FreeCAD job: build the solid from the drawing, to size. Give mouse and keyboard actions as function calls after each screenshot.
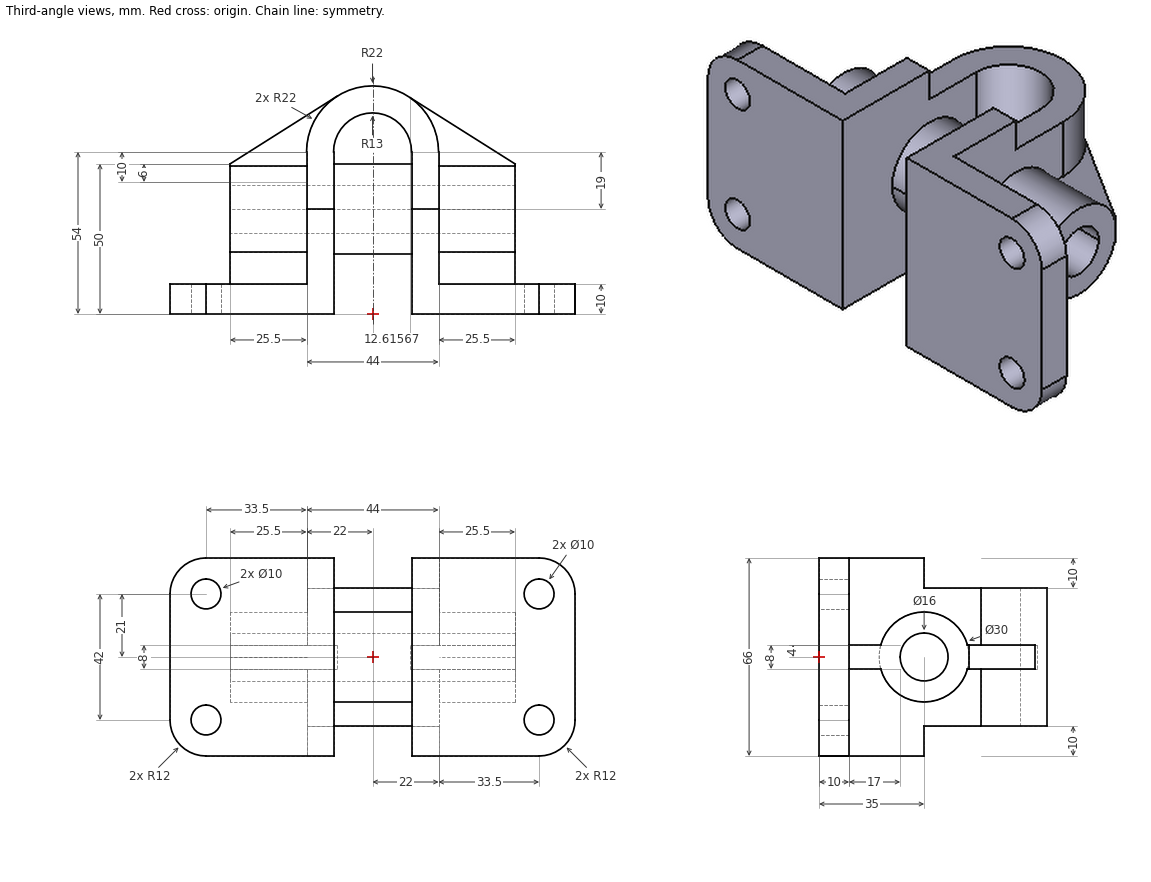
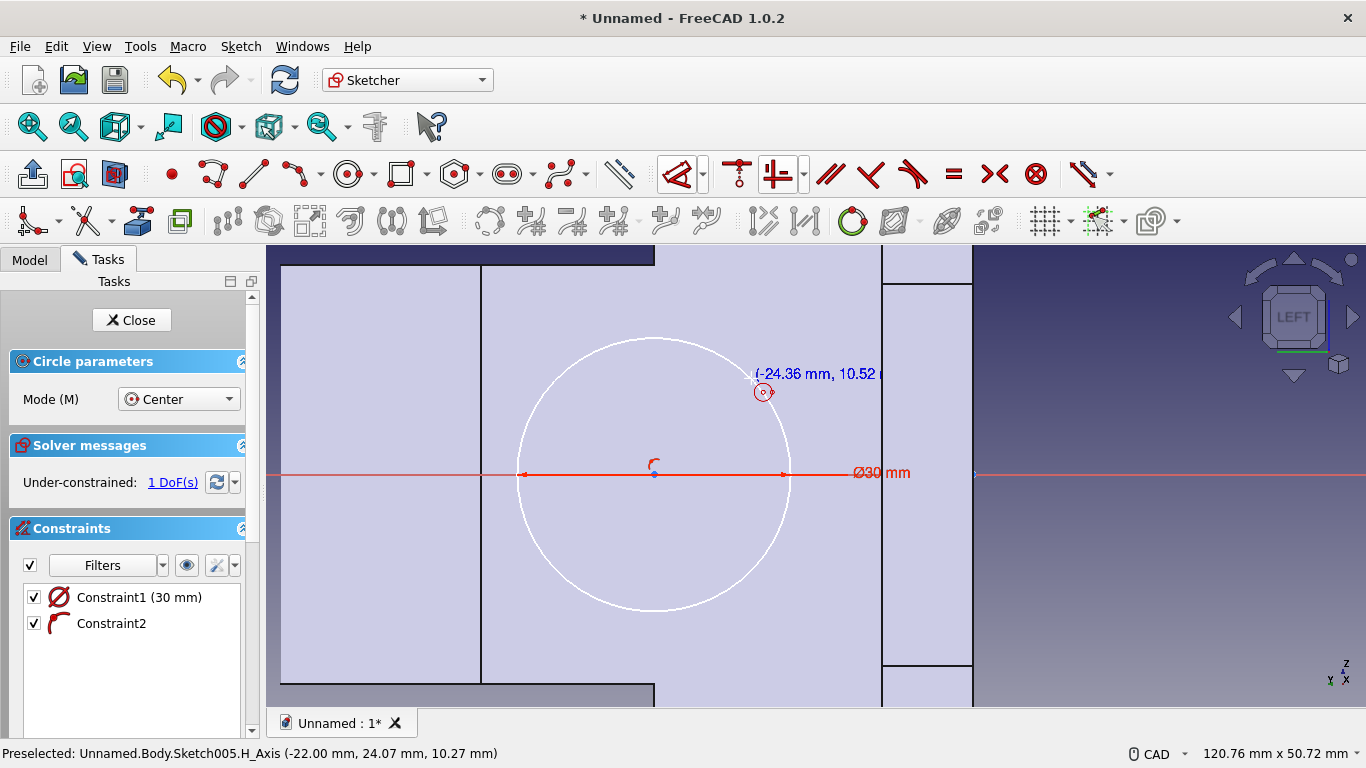
click(654, 475)
move(706, 423)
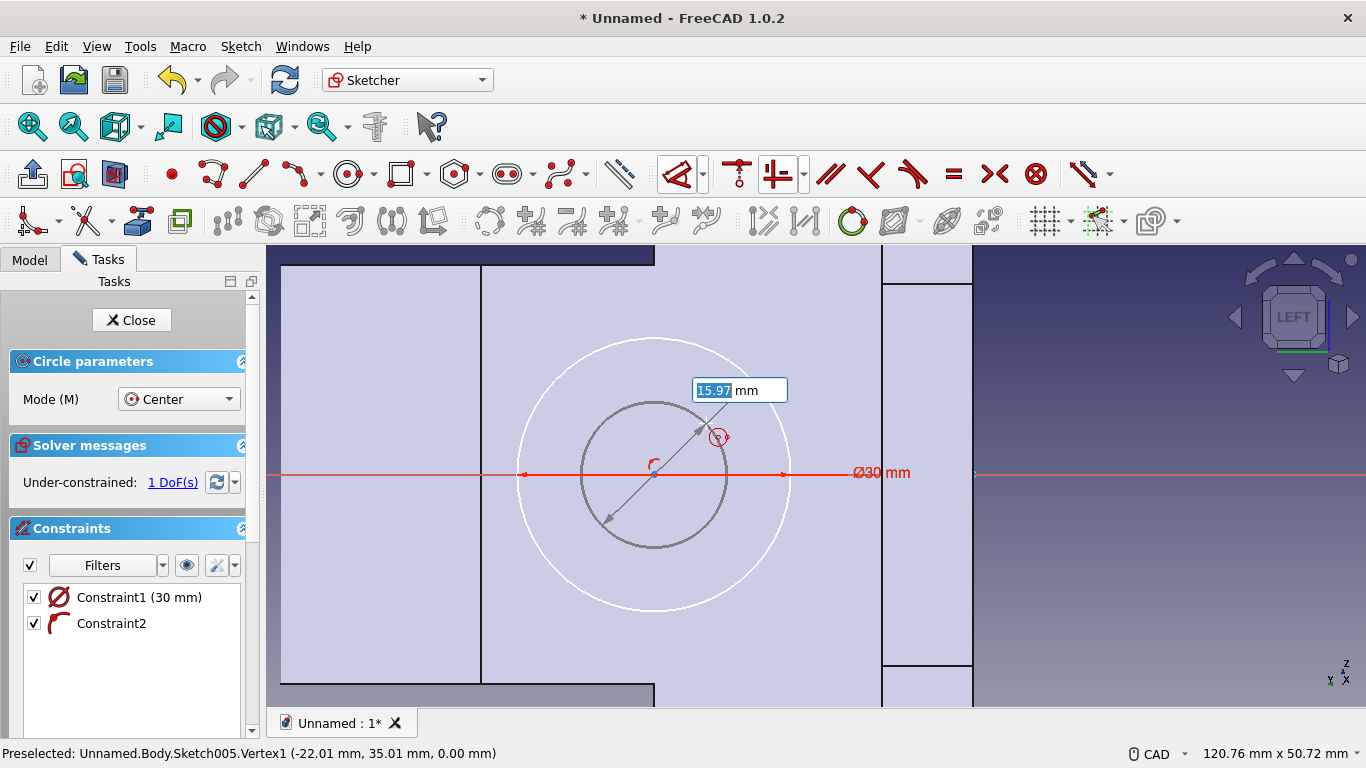
text(16)
key(Return)
key(Escape)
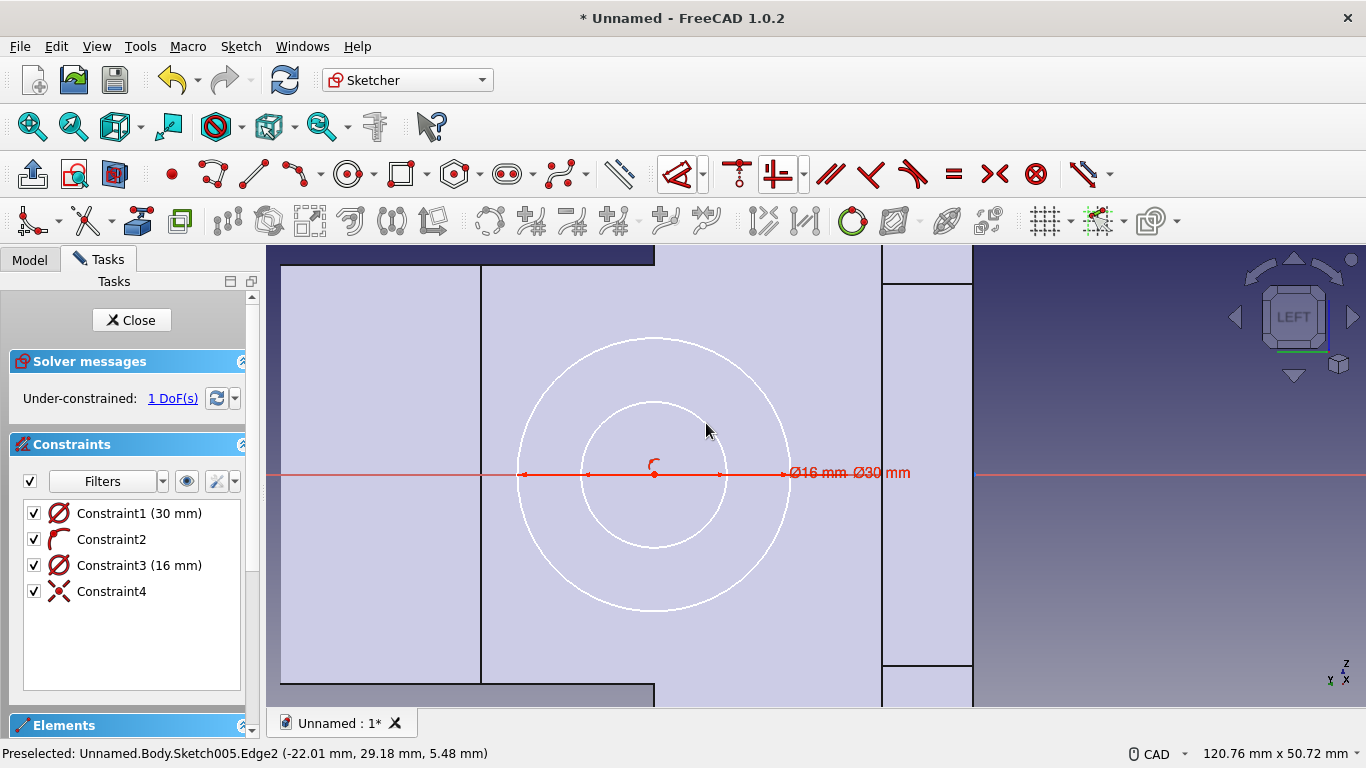
click(654, 475)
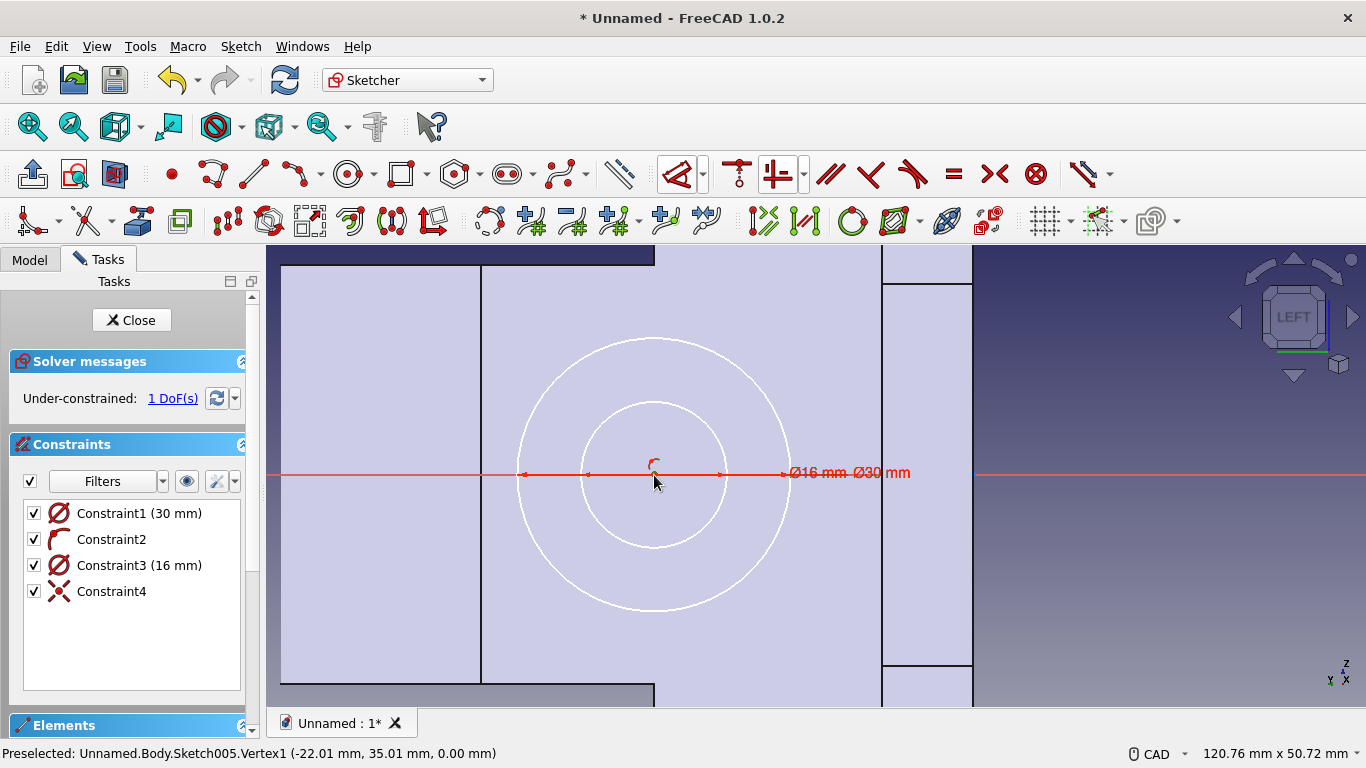
key(l)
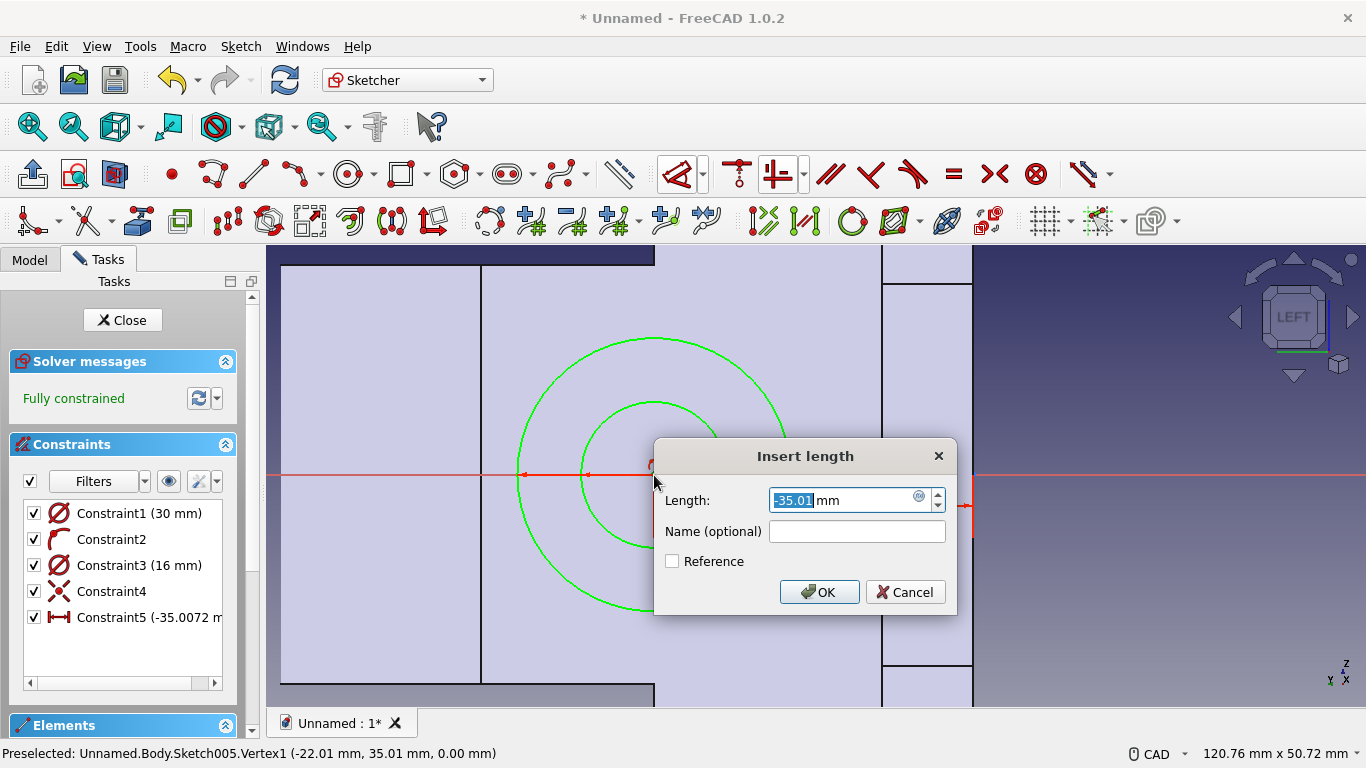
text(-35)
key(Return)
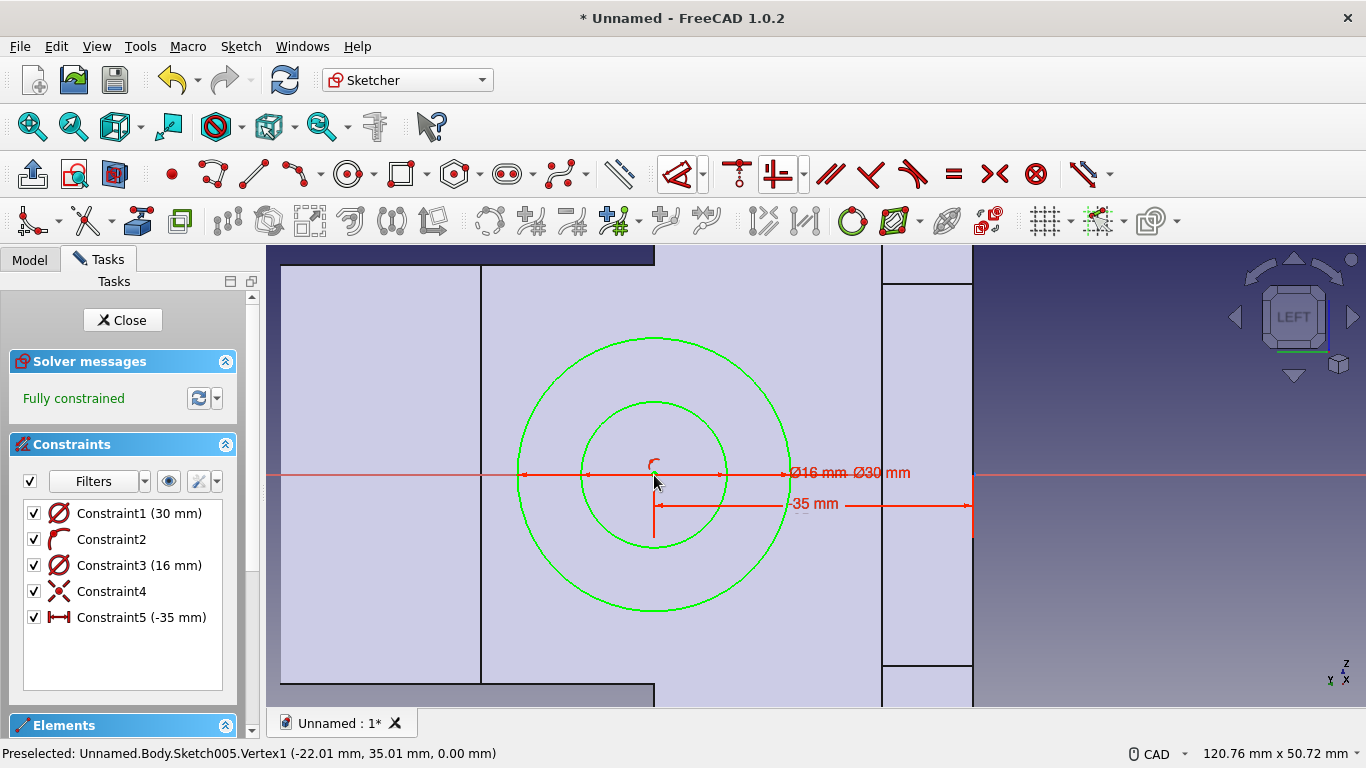
click(123, 320)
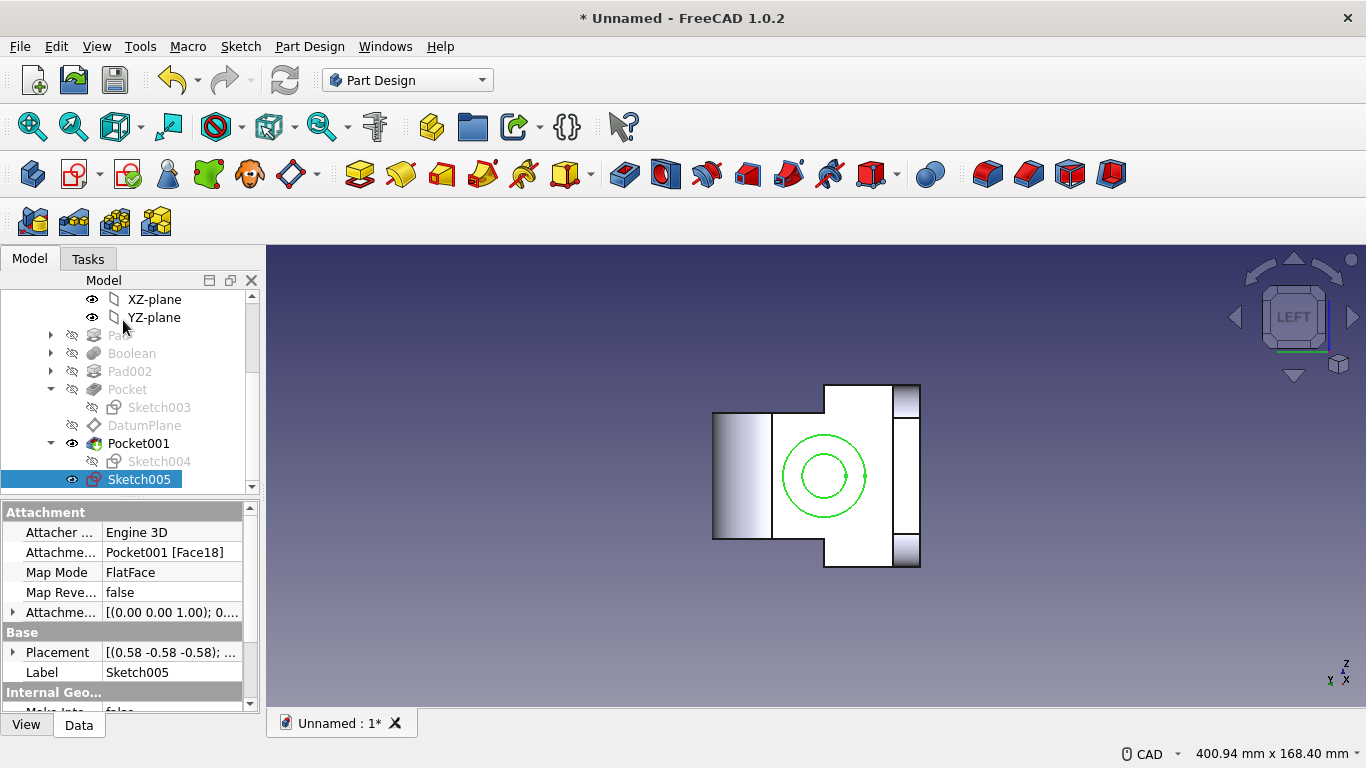
click(360, 174)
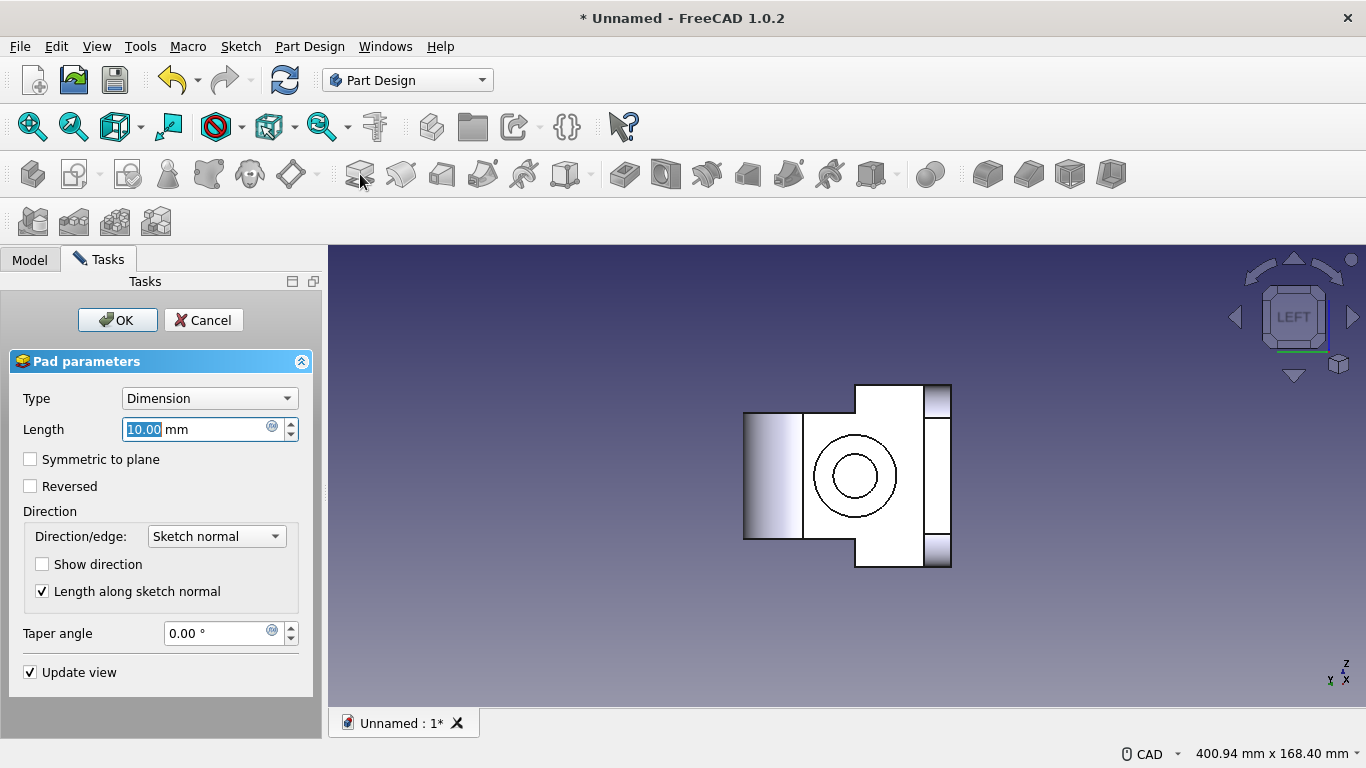
text(44)
key(Tab)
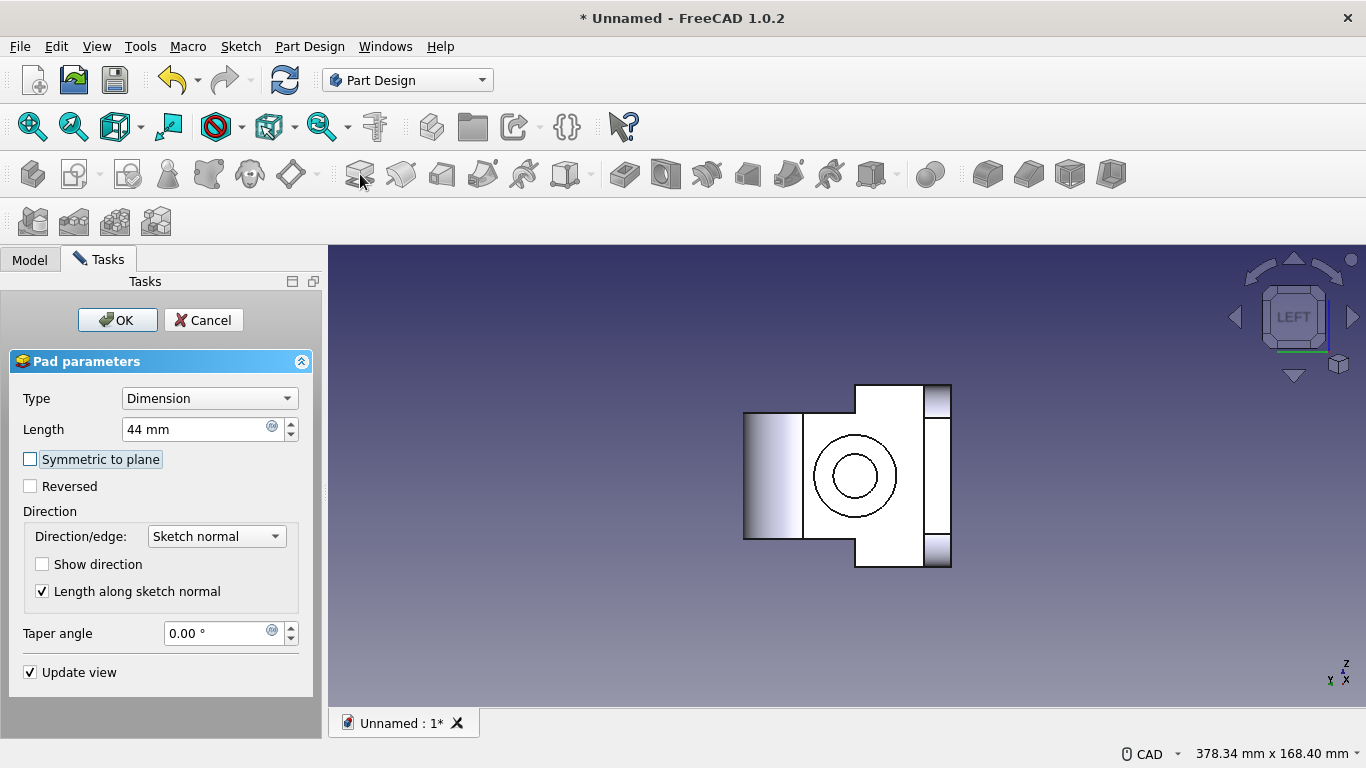
click(31, 486)